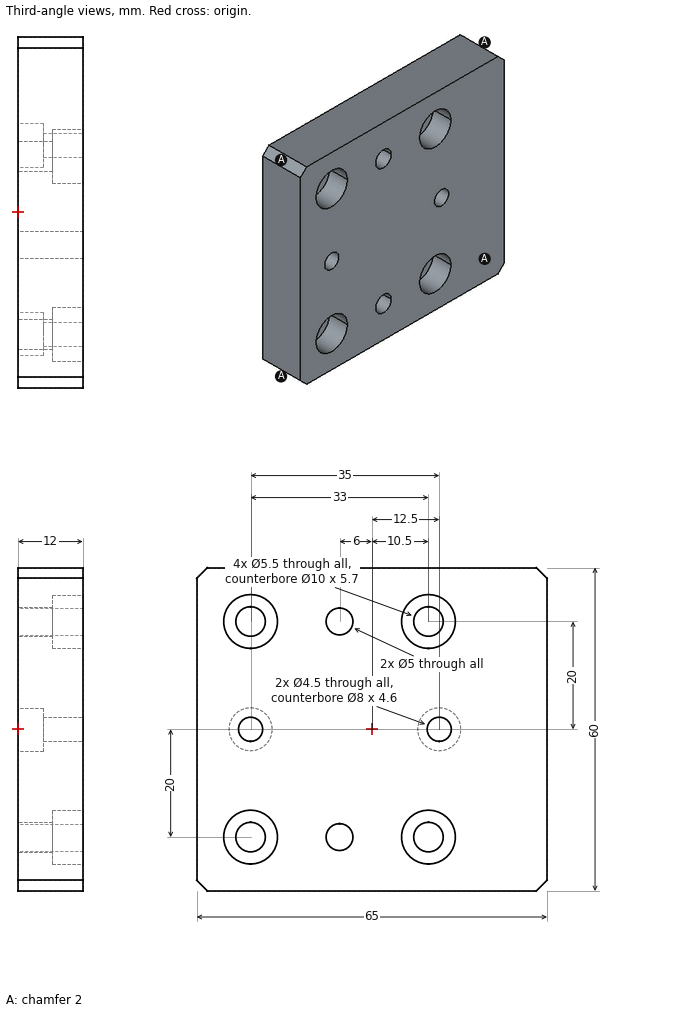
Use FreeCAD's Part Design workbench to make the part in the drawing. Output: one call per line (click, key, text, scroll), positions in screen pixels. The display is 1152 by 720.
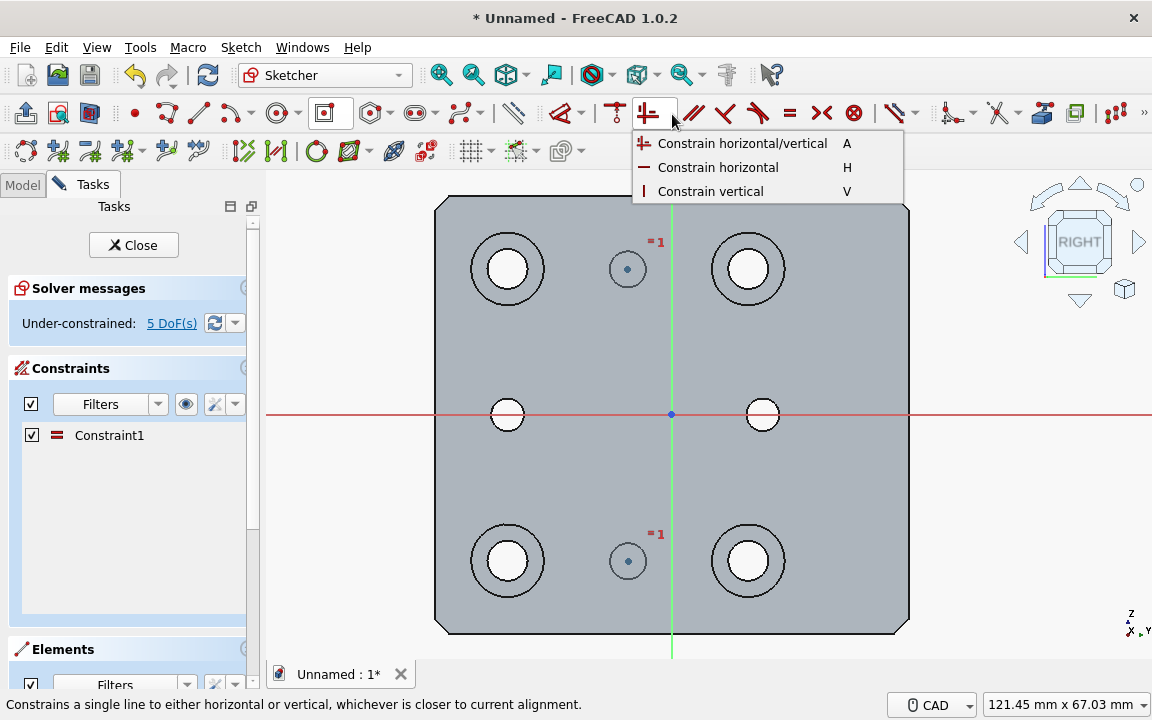
click(768, 191)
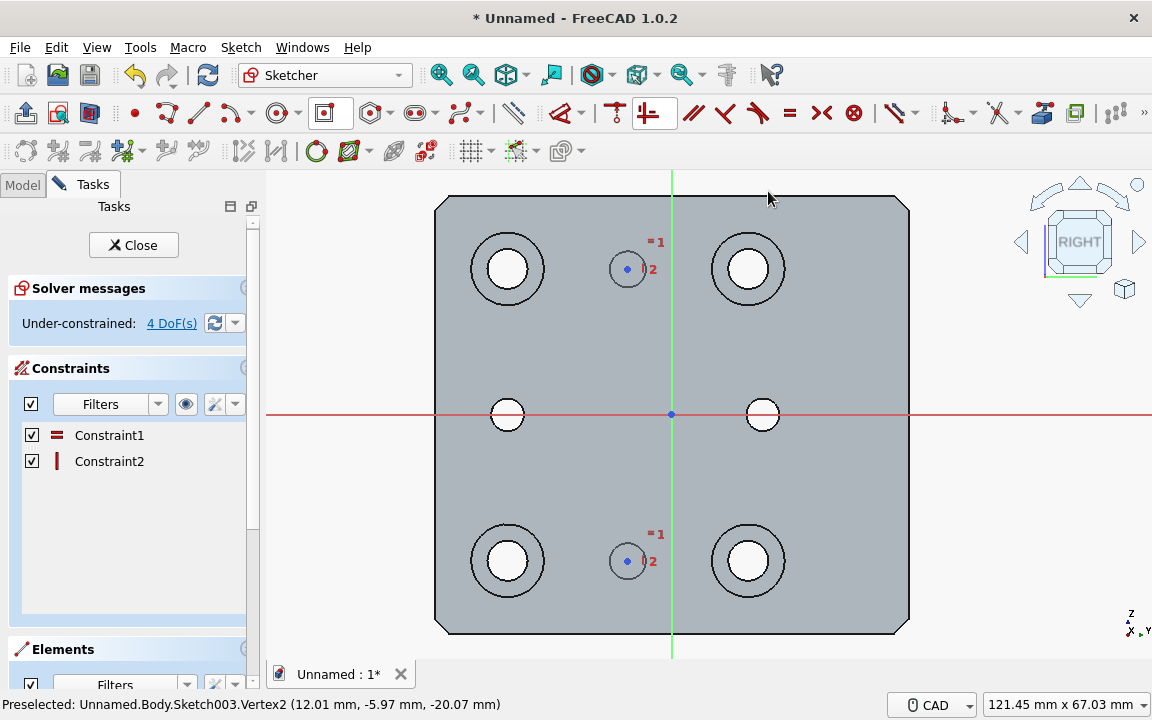
click(560, 114)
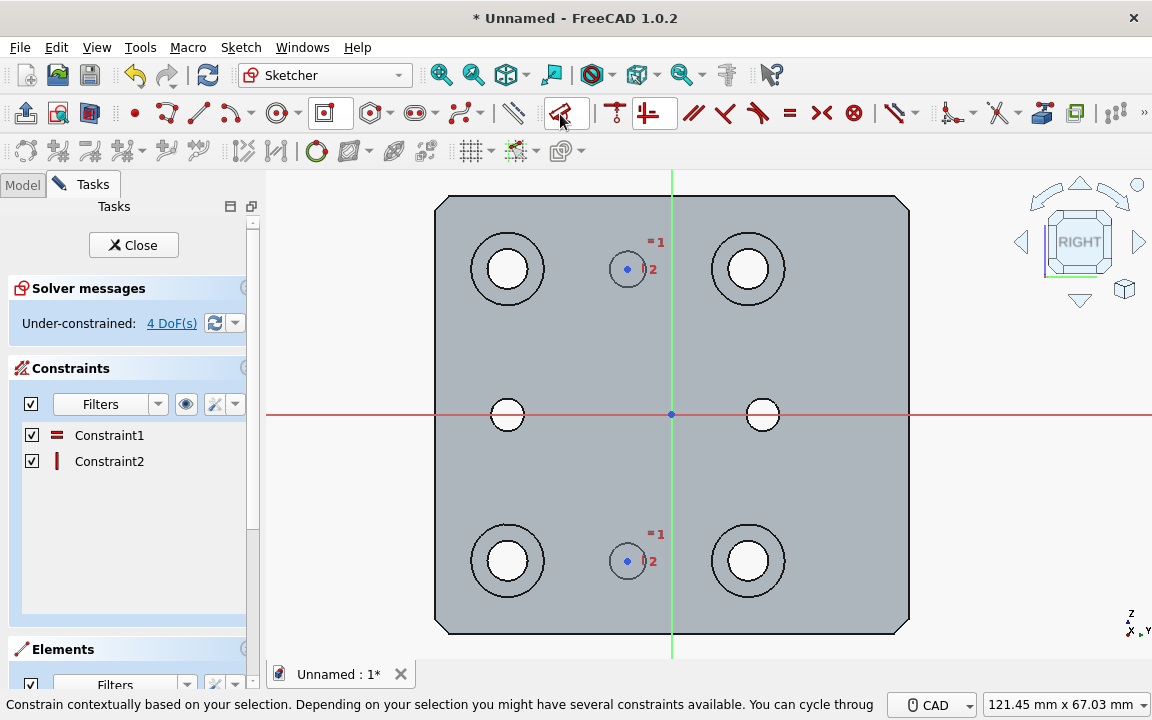
click(640, 257)
click(641, 222)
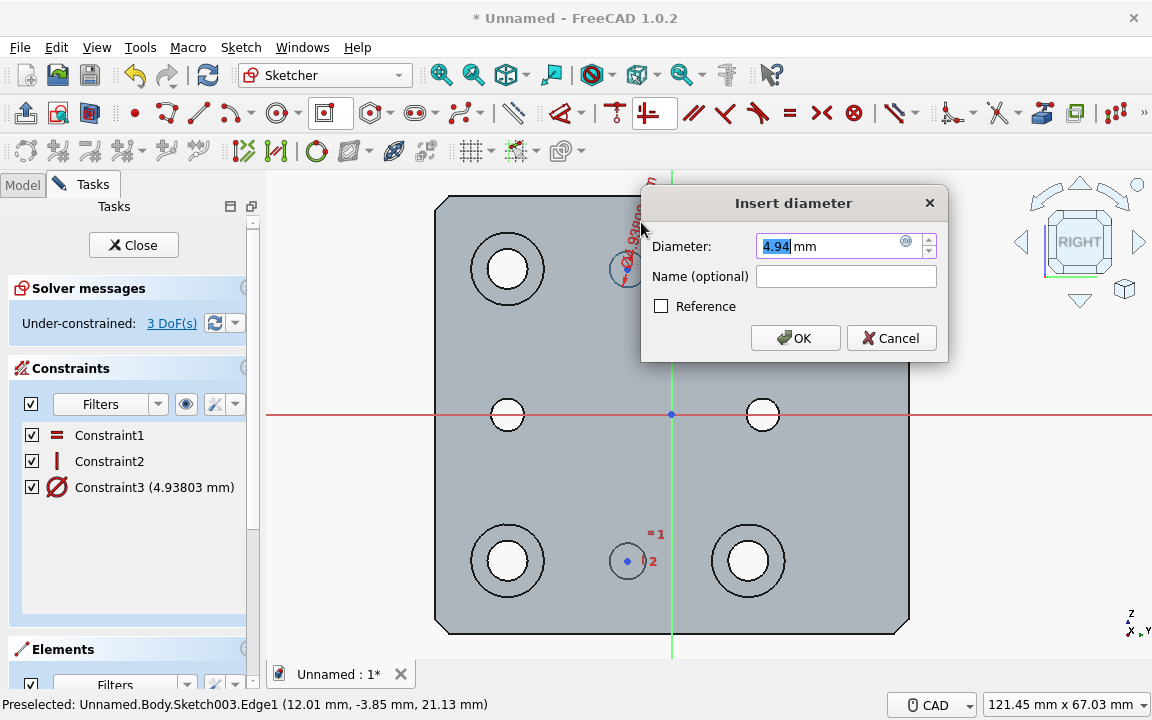
text(5)
key(Return)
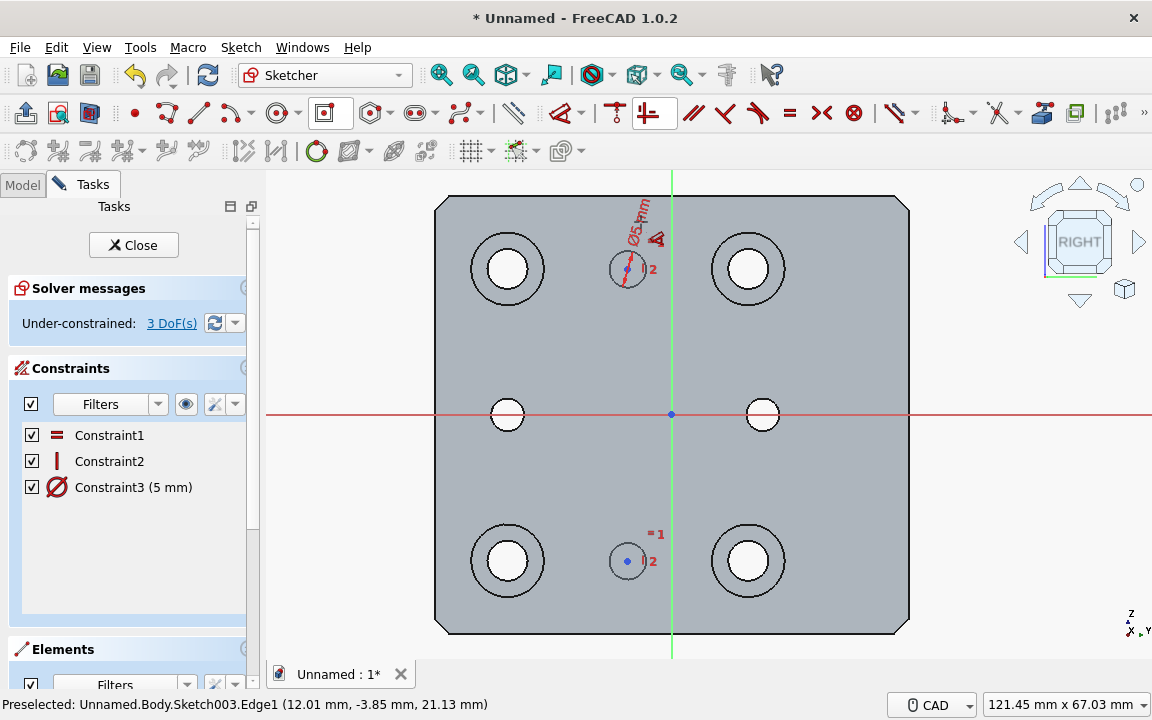
click(628, 269)
click(650, 449)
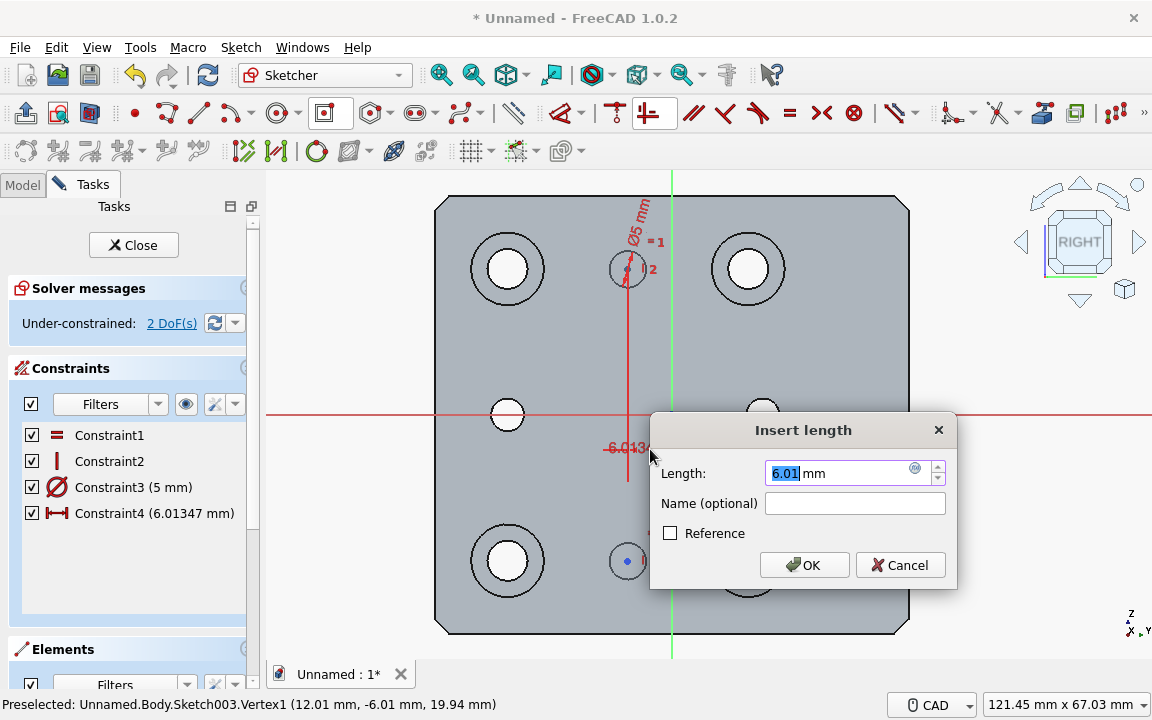
text(6)
key(Return)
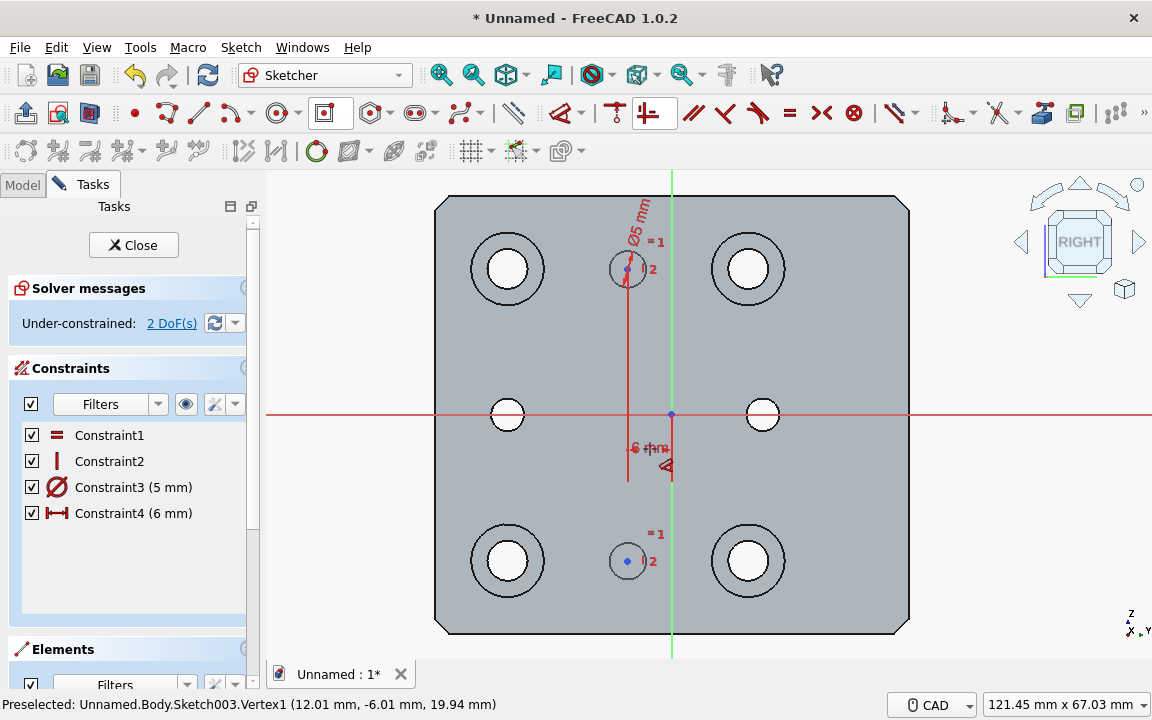
click(628, 269)
click(706, 342)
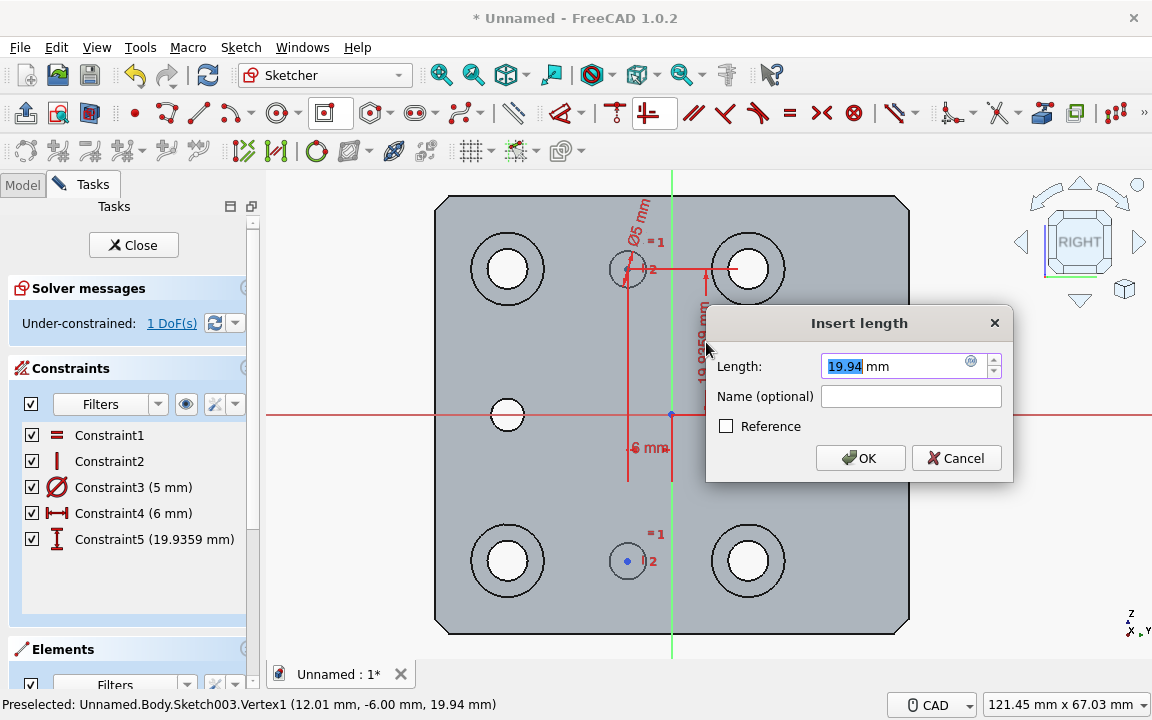
text(20)
key(Return)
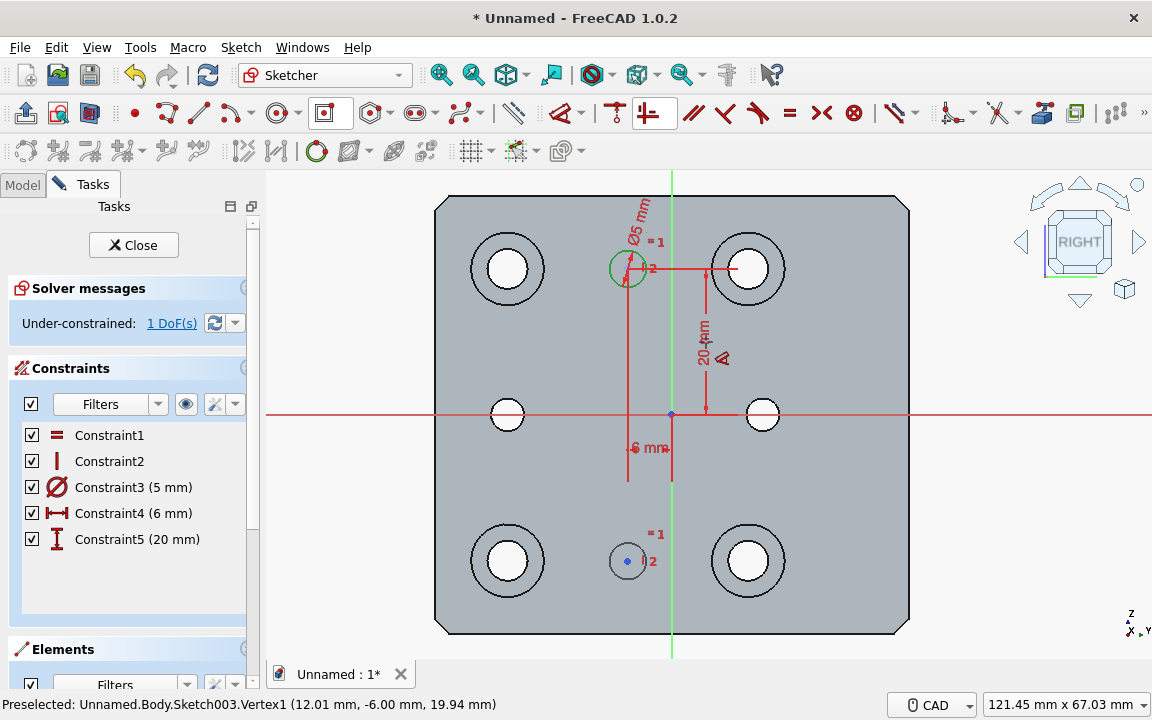
click(628, 561)
click(706, 488)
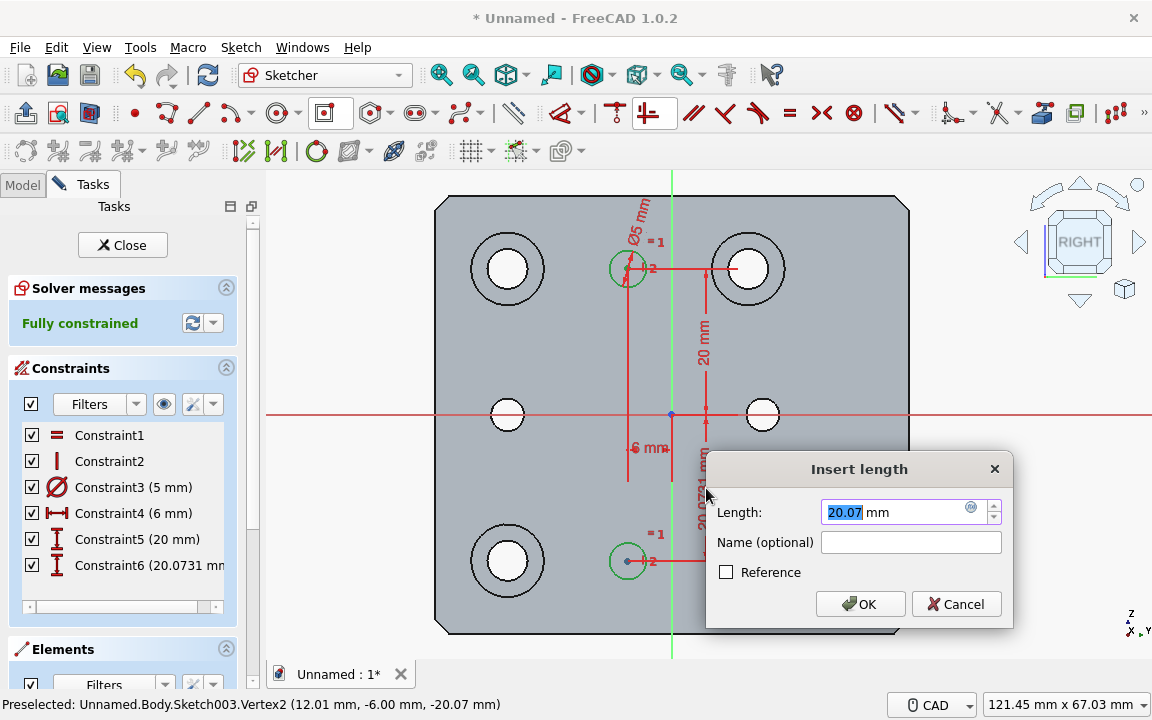
text(20)
key(Return)
key(Escape)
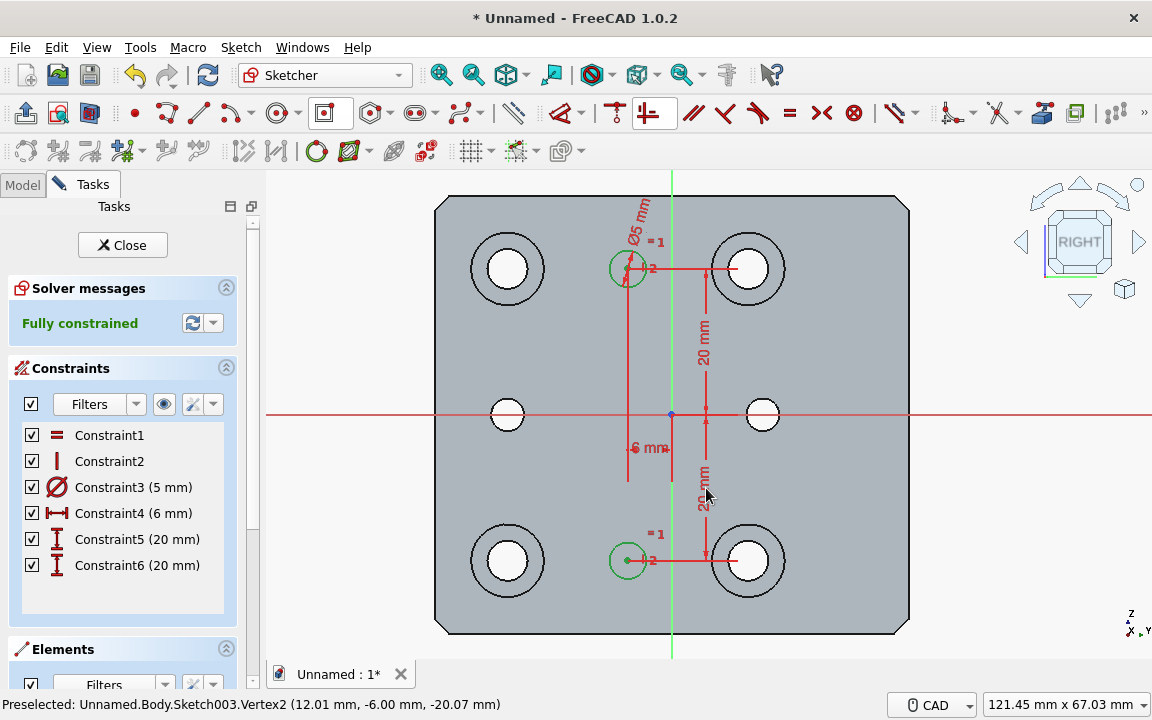
click(123, 245)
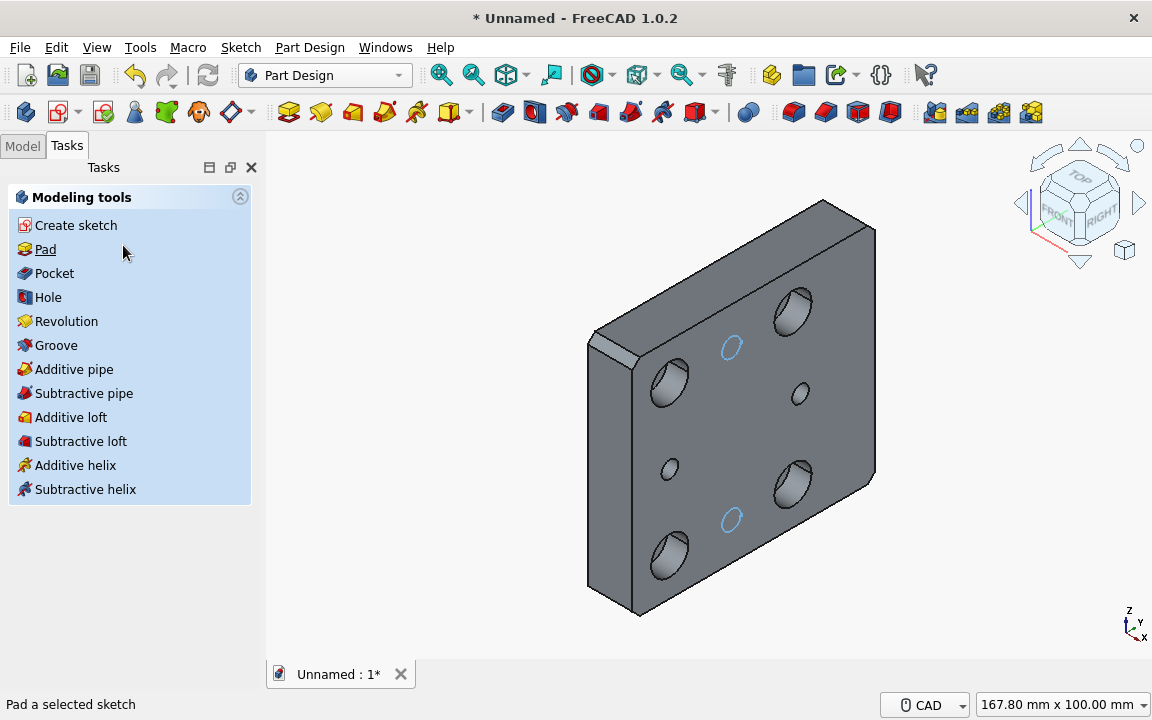
click(536, 112)